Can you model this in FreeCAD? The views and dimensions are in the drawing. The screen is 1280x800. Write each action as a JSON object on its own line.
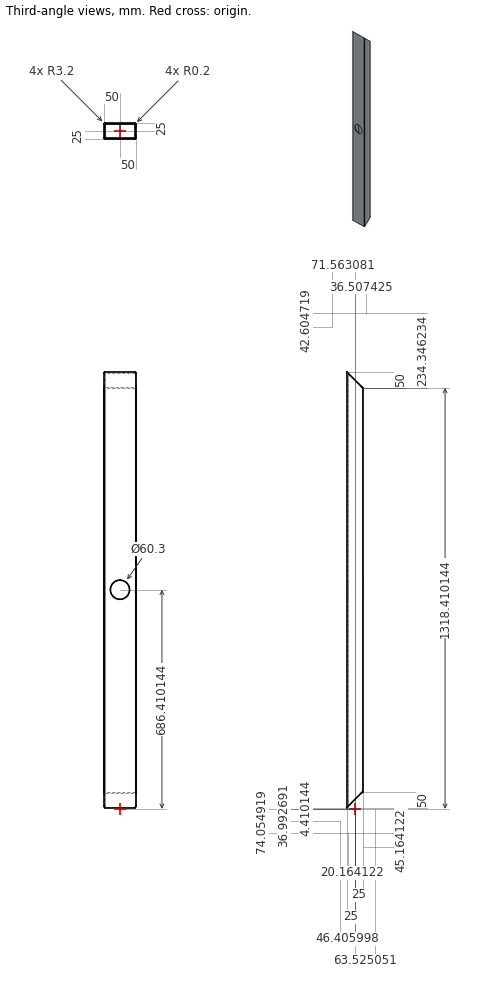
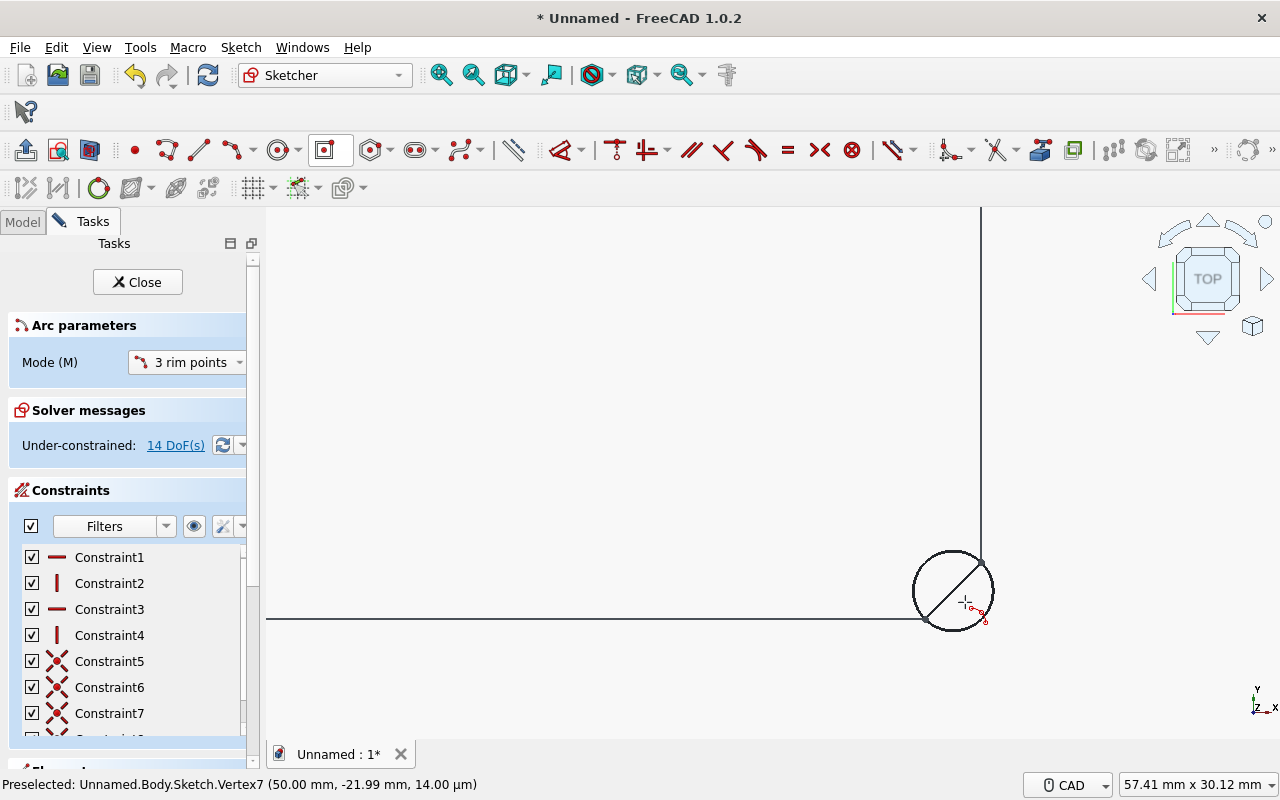
{"action": "left_click", "coordinate": [965, 599]}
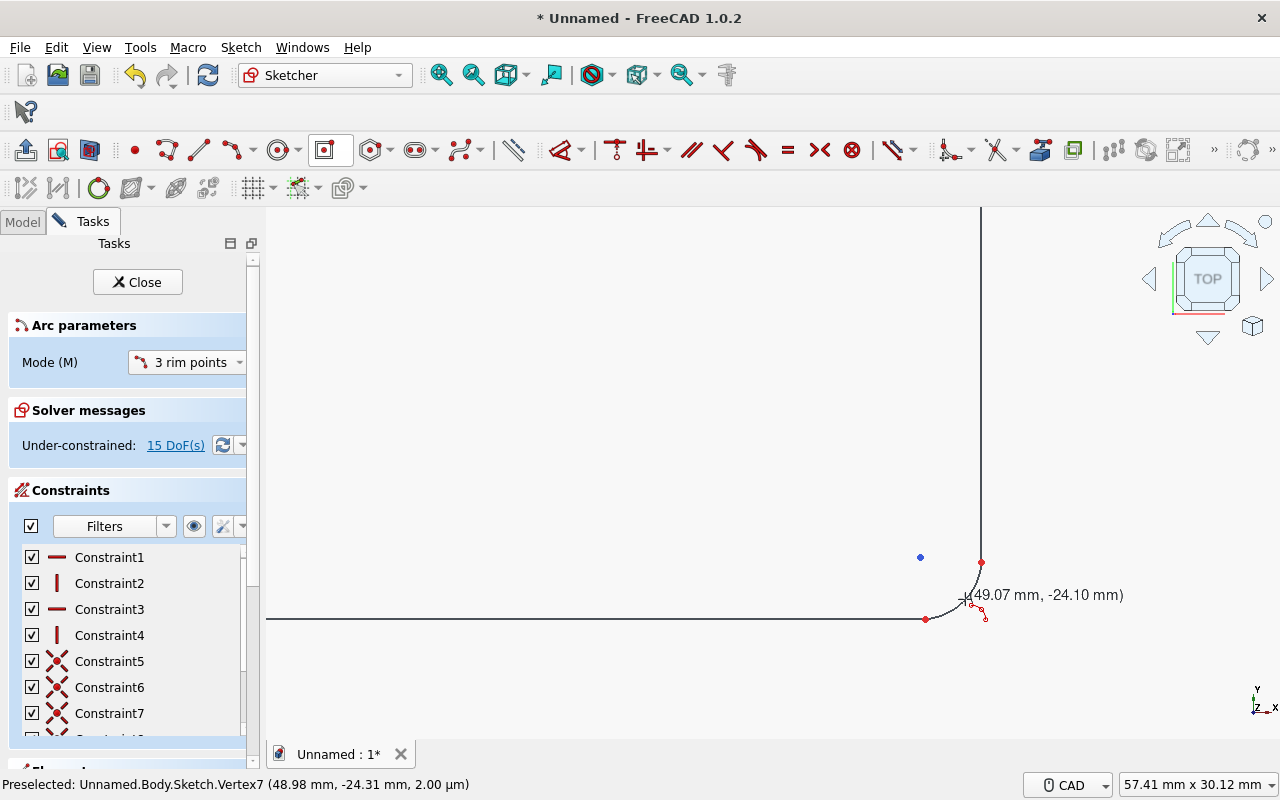
{"action": "scroll", "coordinate": [966, 602], "scroll_direction": "down", "scroll_amount": 6}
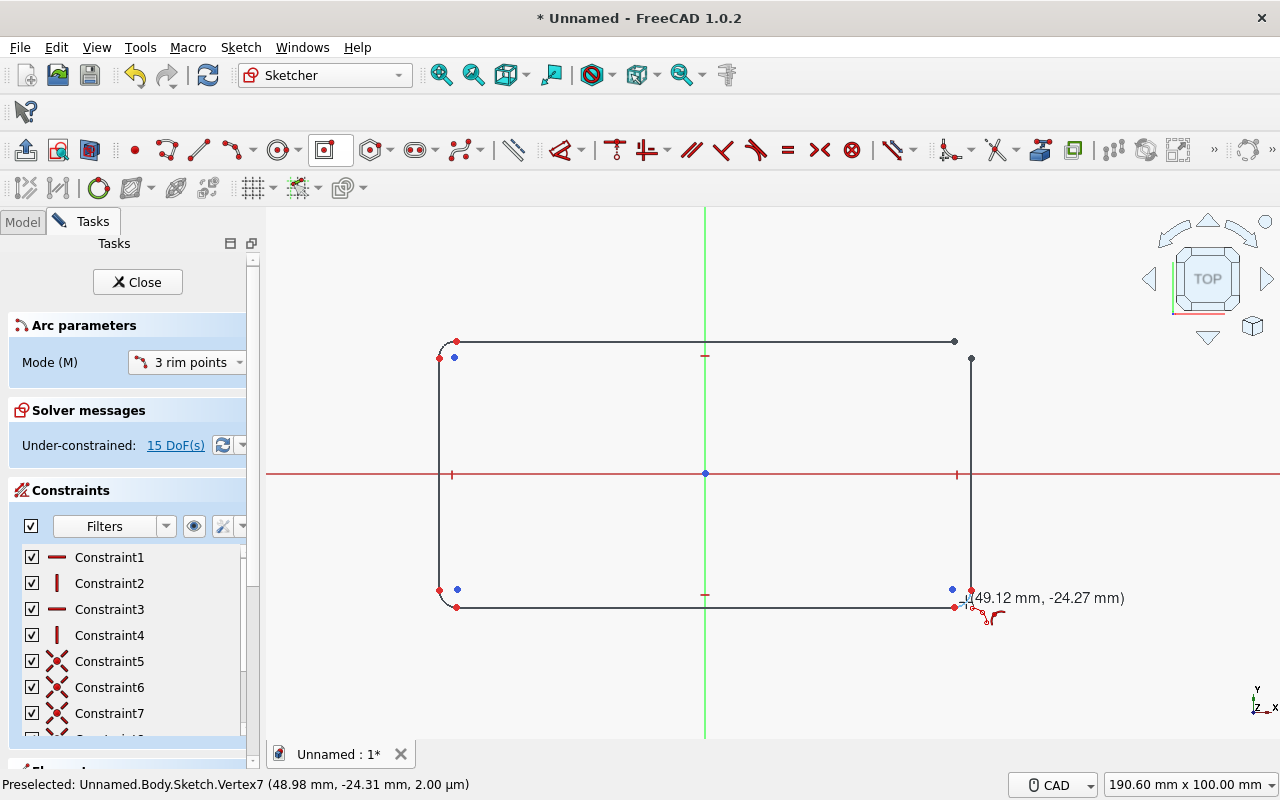
{"action": "left_click", "coordinate": [971, 359]}
{"action": "left_click", "coordinate": [954, 342]}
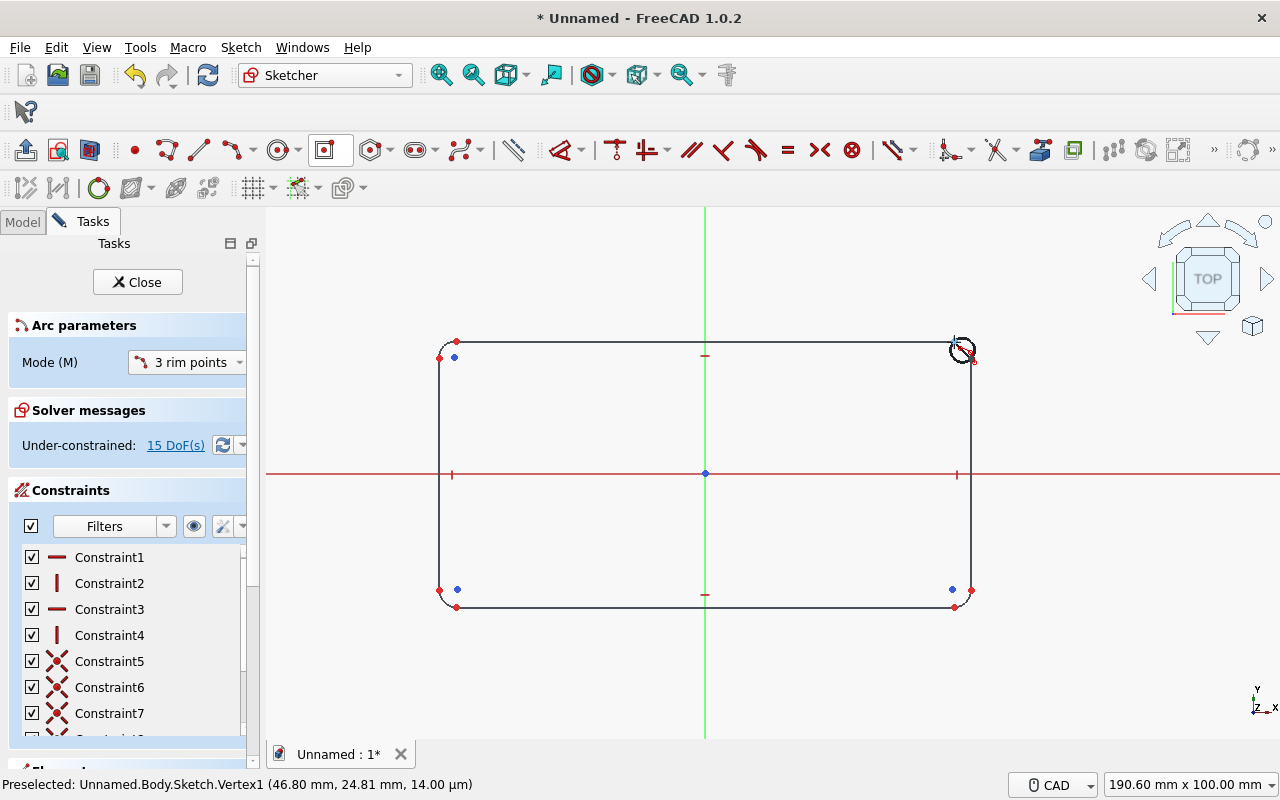
{"action": "scroll", "coordinate": [966, 346], "scroll_direction": "up", "scroll_amount": 6}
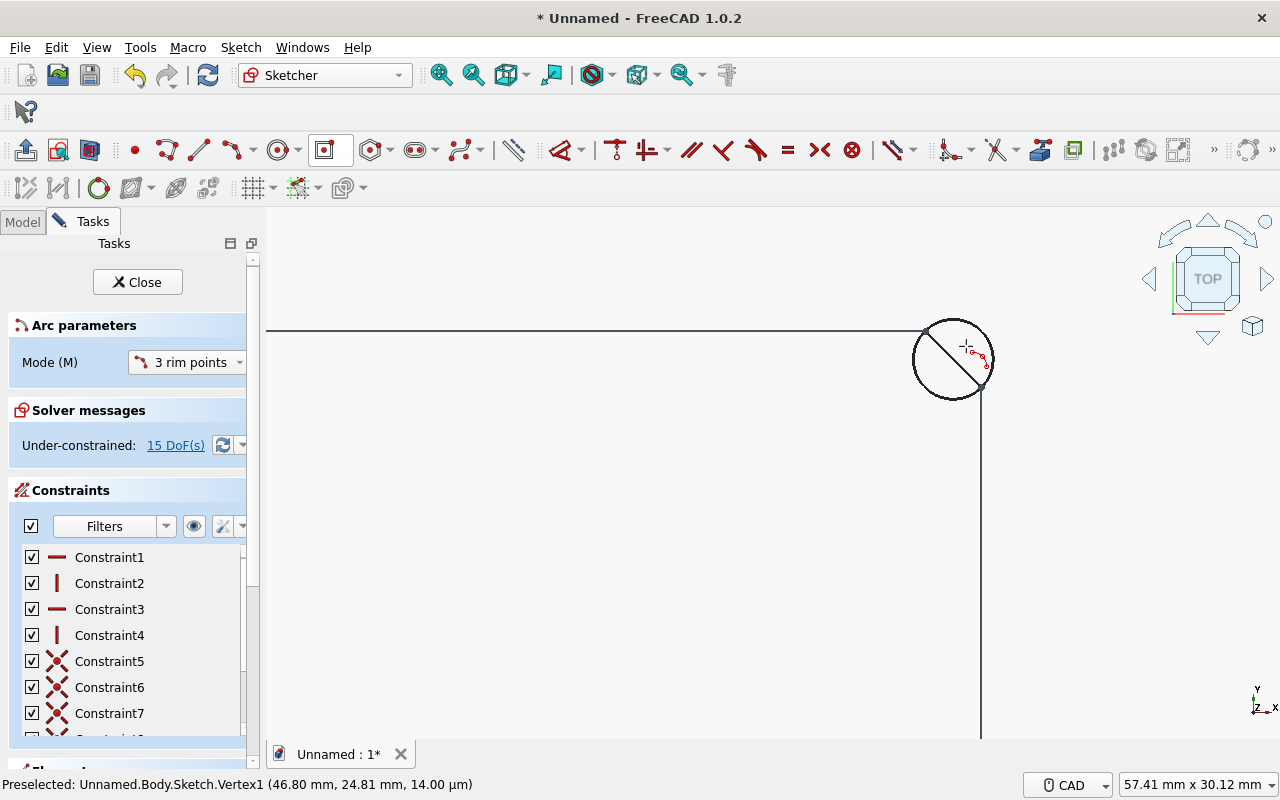
{"action": "left_click", "coordinate": [965, 344]}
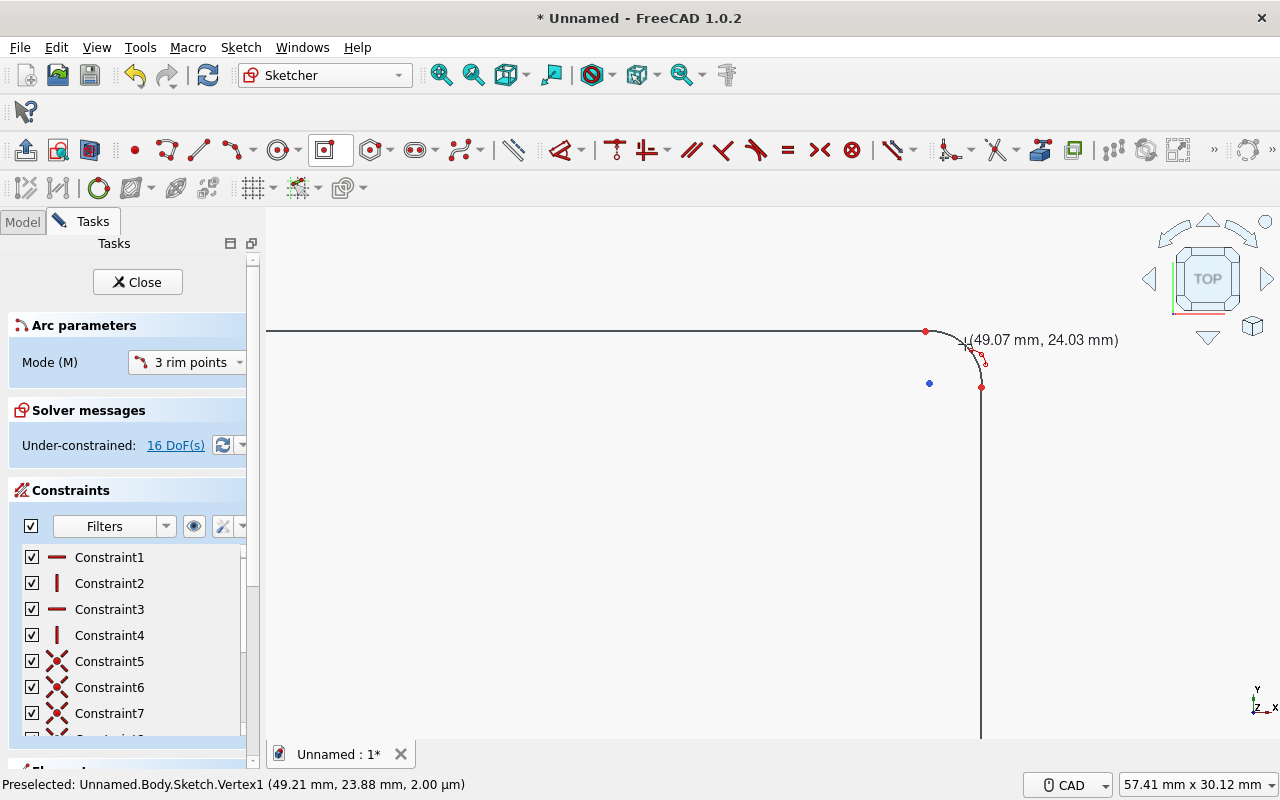
{"action": "left_click", "coordinate": [200, 150]}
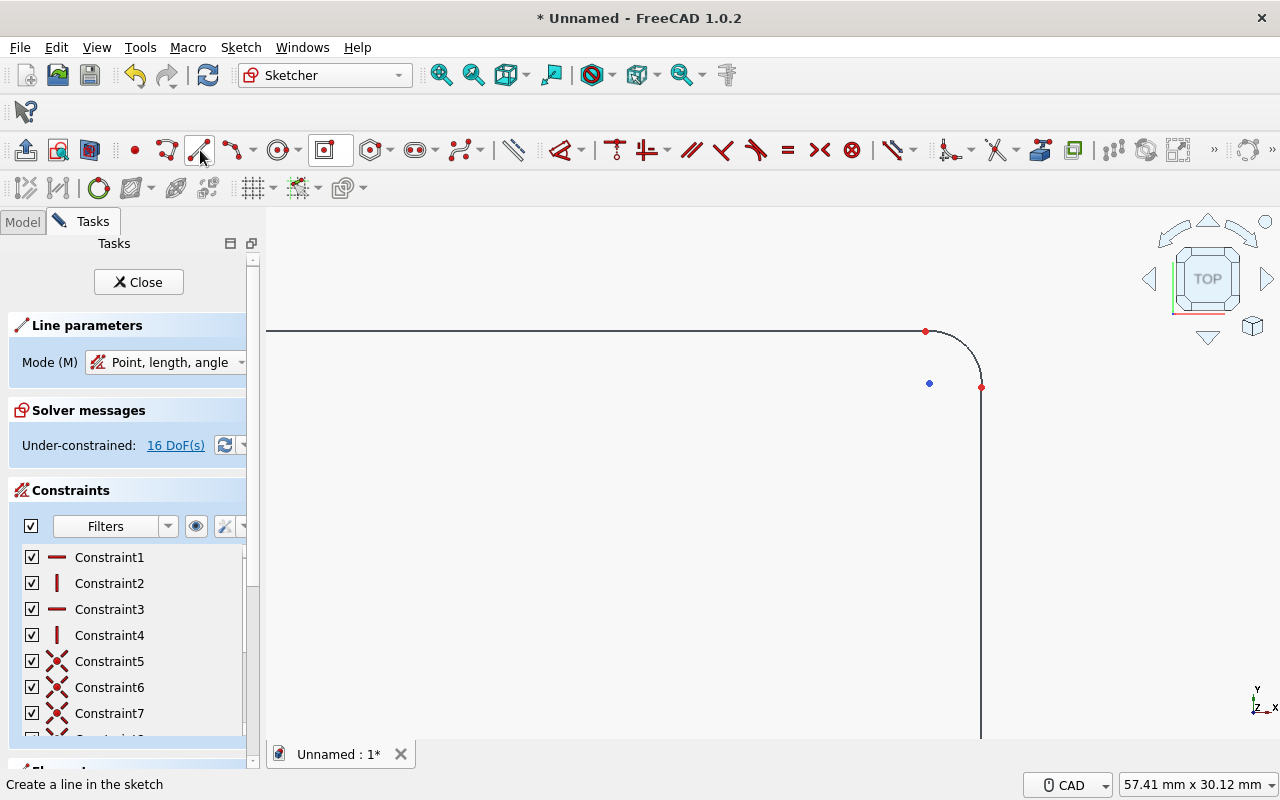
{"action": "scroll", "coordinate": [966, 345], "scroll_direction": "down", "scroll_amount": 6}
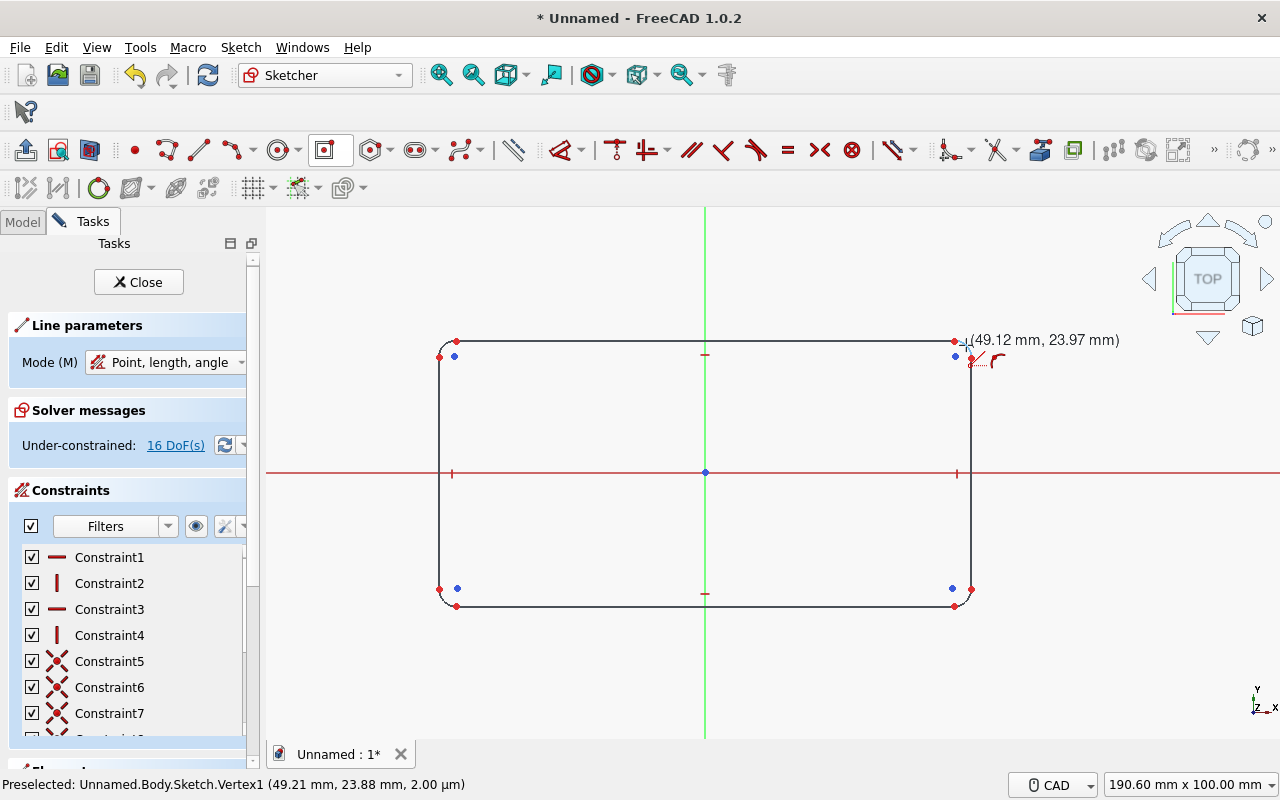
{"action": "scroll", "coordinate": [456, 356], "scroll_direction": "up", "scroll_amount": 14}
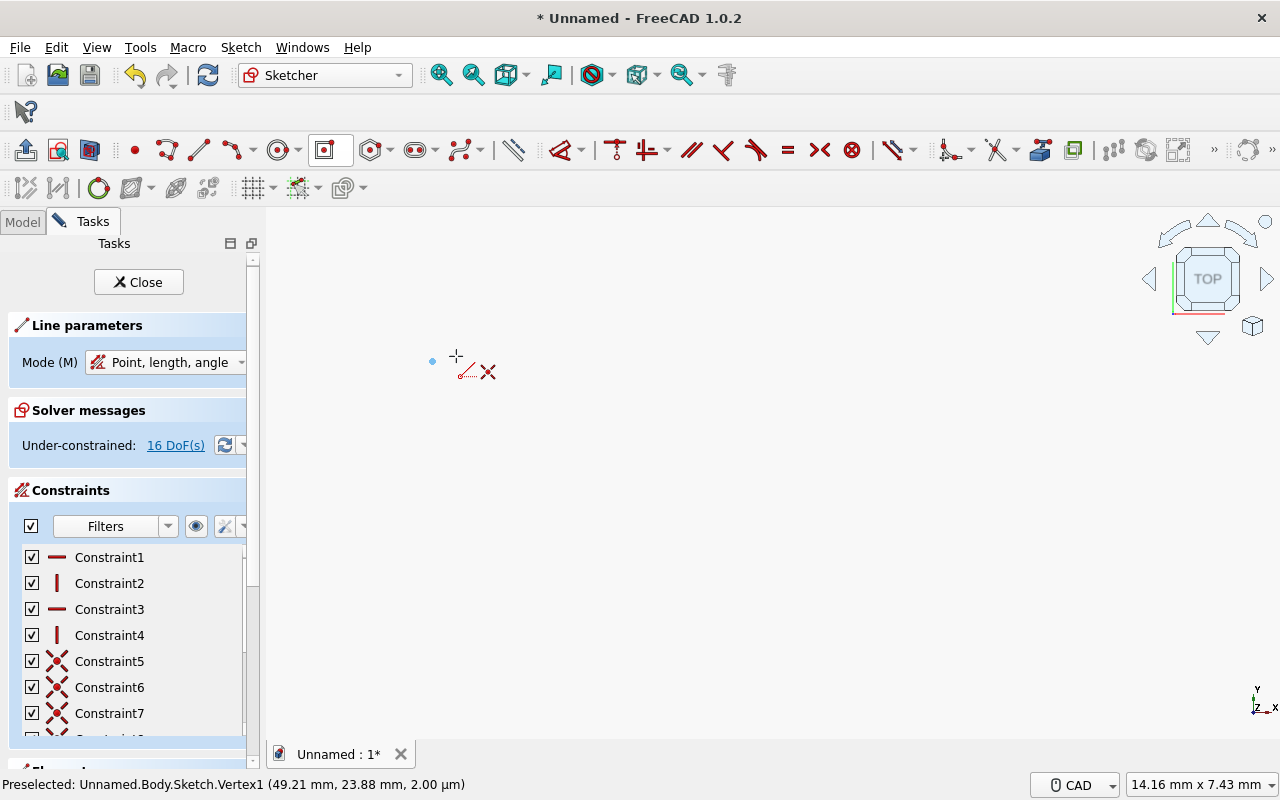
{"action": "left_click", "coordinate": [456, 351]}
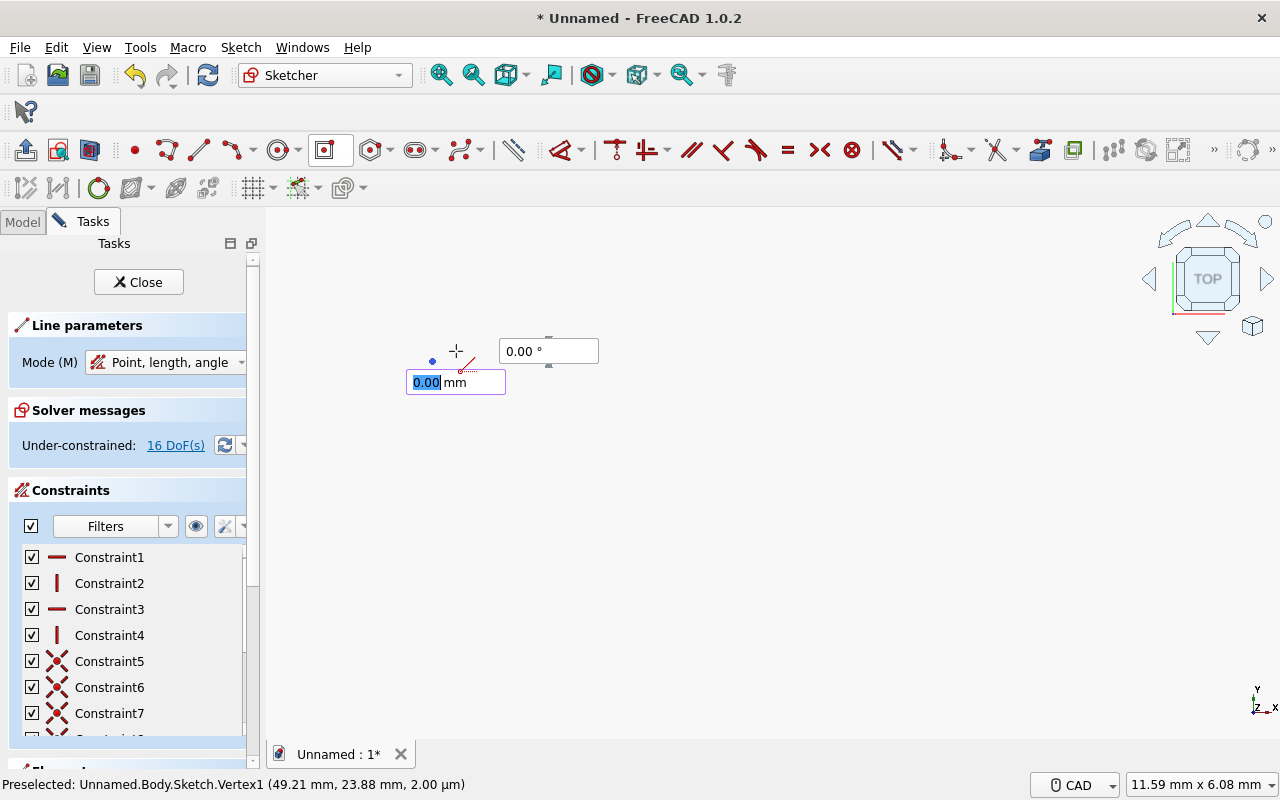
{"action": "scroll", "coordinate": [455, 356], "scroll_direction": "down", "scroll_amount": 14}